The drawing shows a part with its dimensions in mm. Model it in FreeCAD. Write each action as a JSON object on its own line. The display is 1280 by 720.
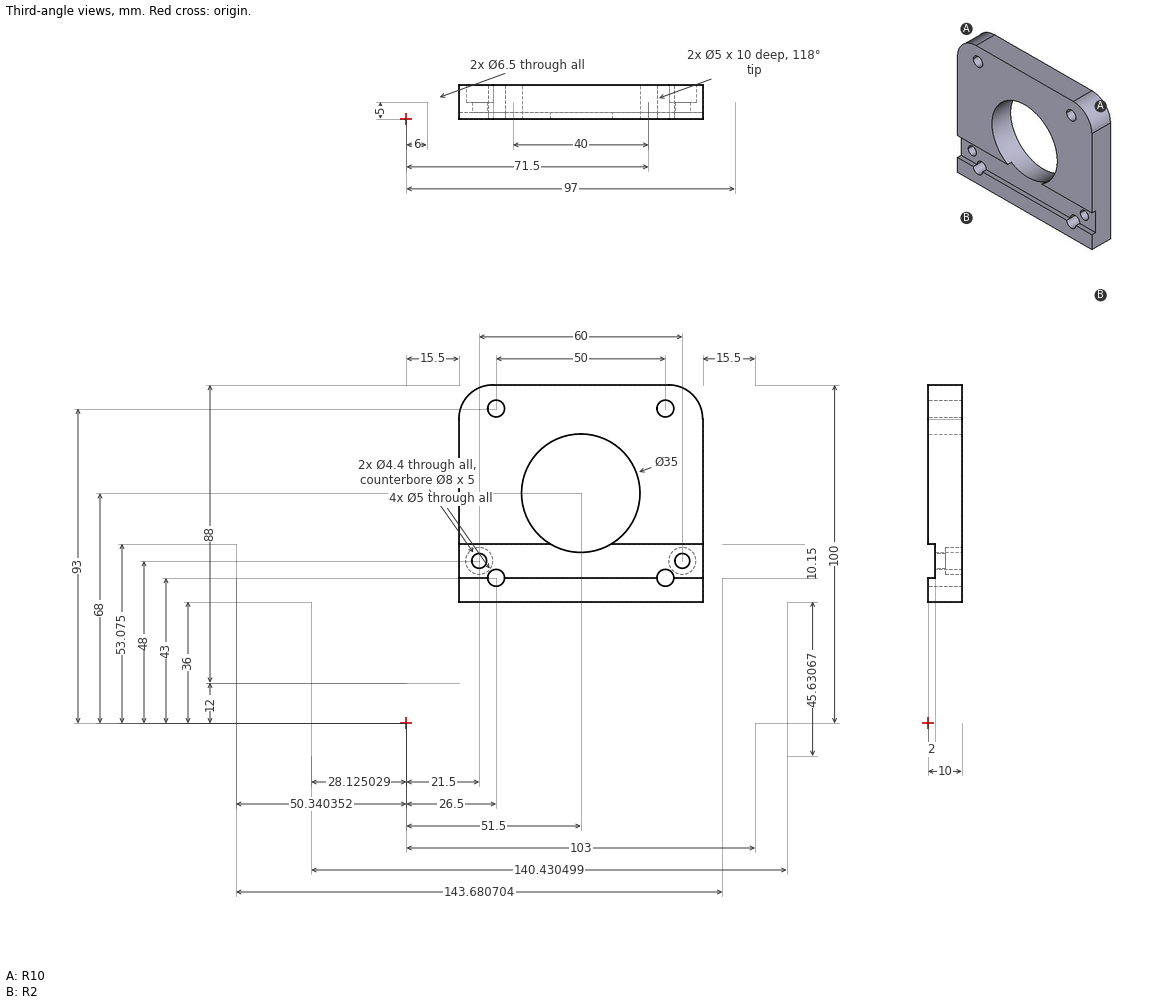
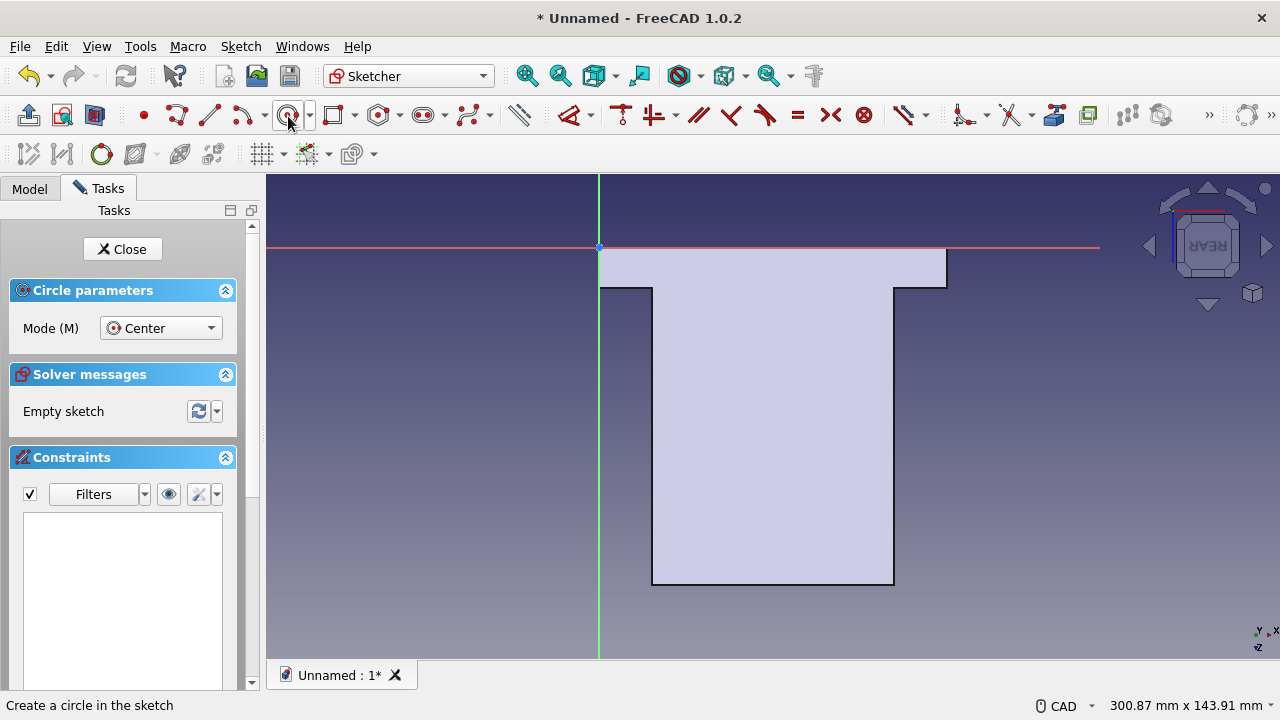
{"action": "left_click", "coordinate": [773, 477]}
{"action": "mouse_move", "coordinate": [815, 435]}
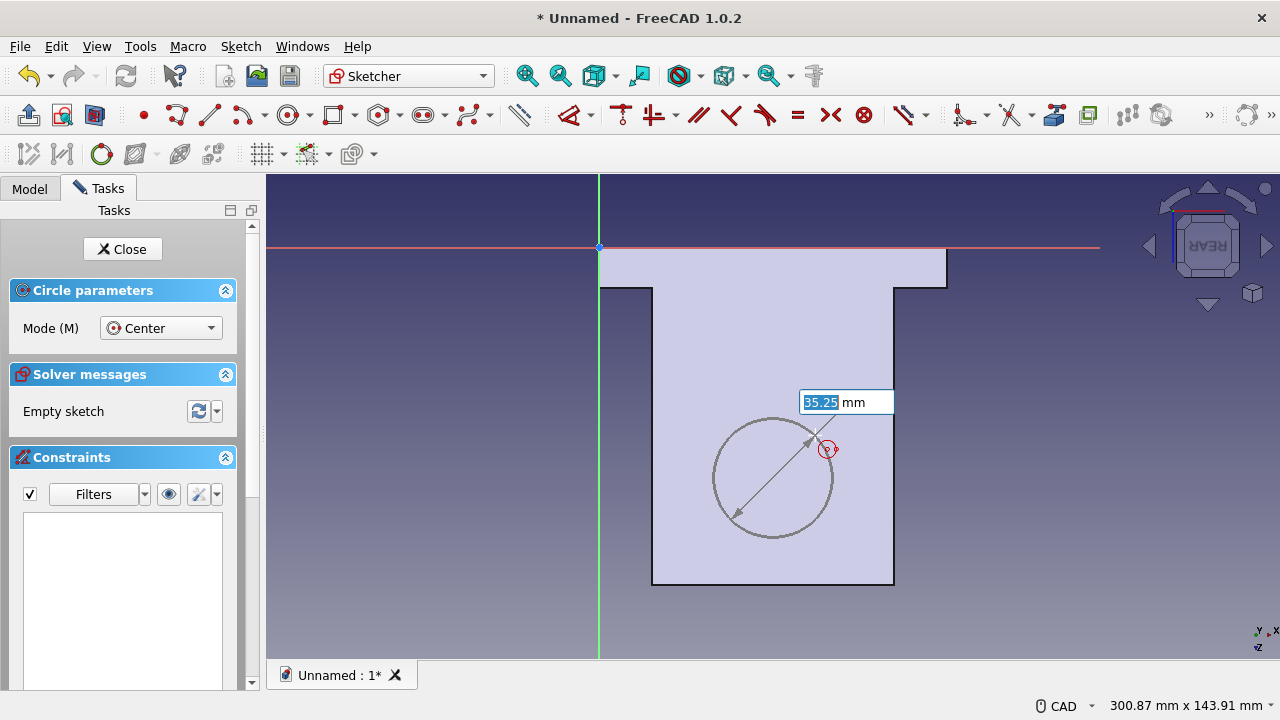
{"action": "type", "text": "35"}
{"action": "key", "text": "Return"}
{"action": "key", "text": "Escape"}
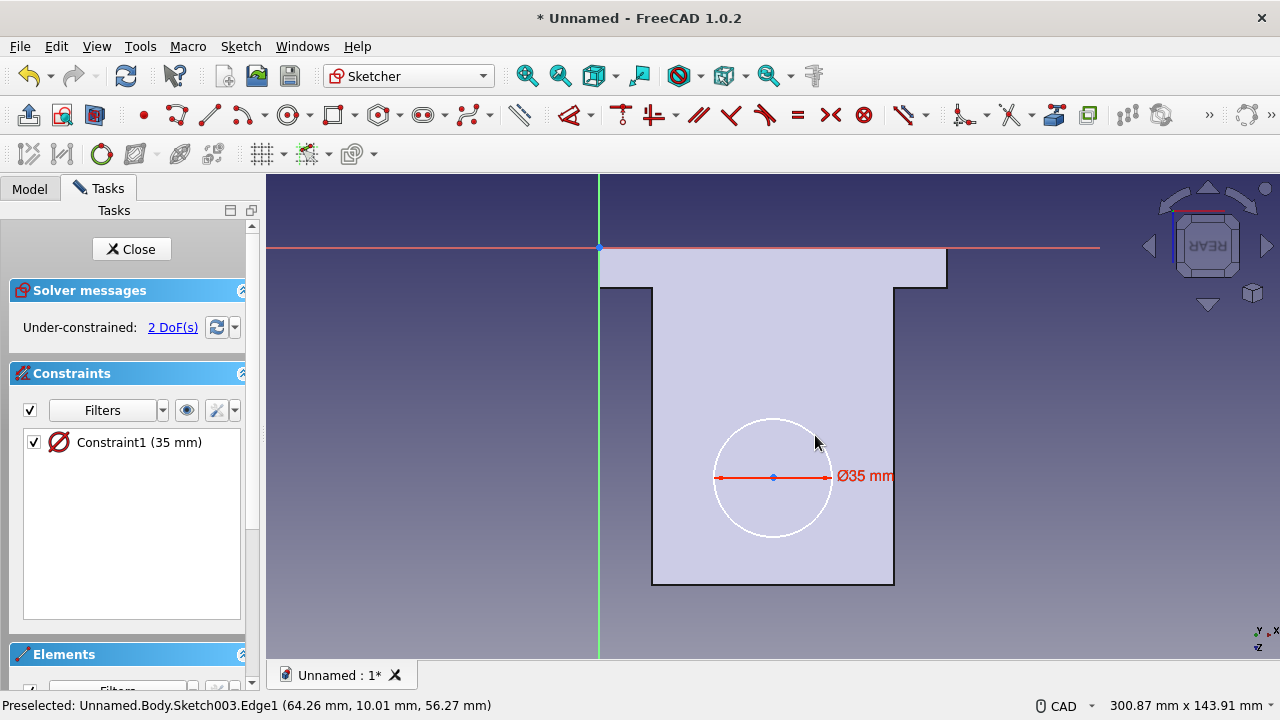
{"action": "left_click", "coordinate": [568, 116]}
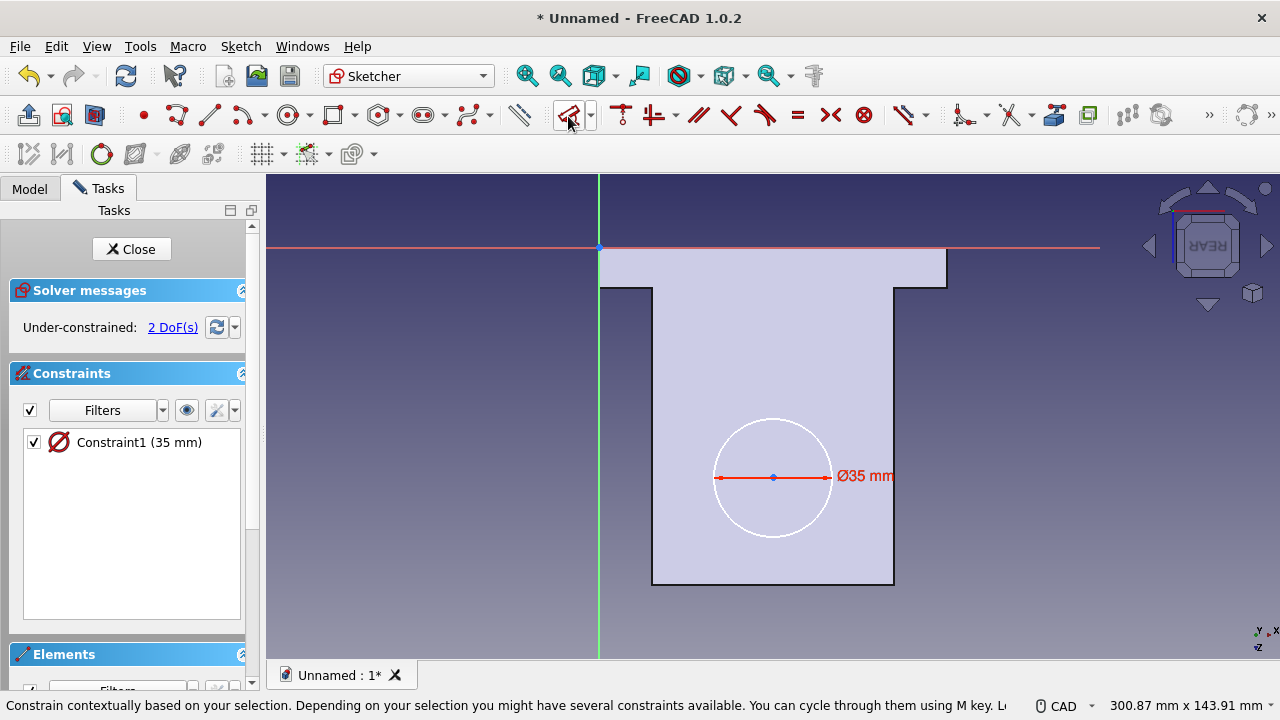
{"action": "left_click", "coordinate": [773, 478]}
{"action": "left_click", "coordinate": [565, 363]}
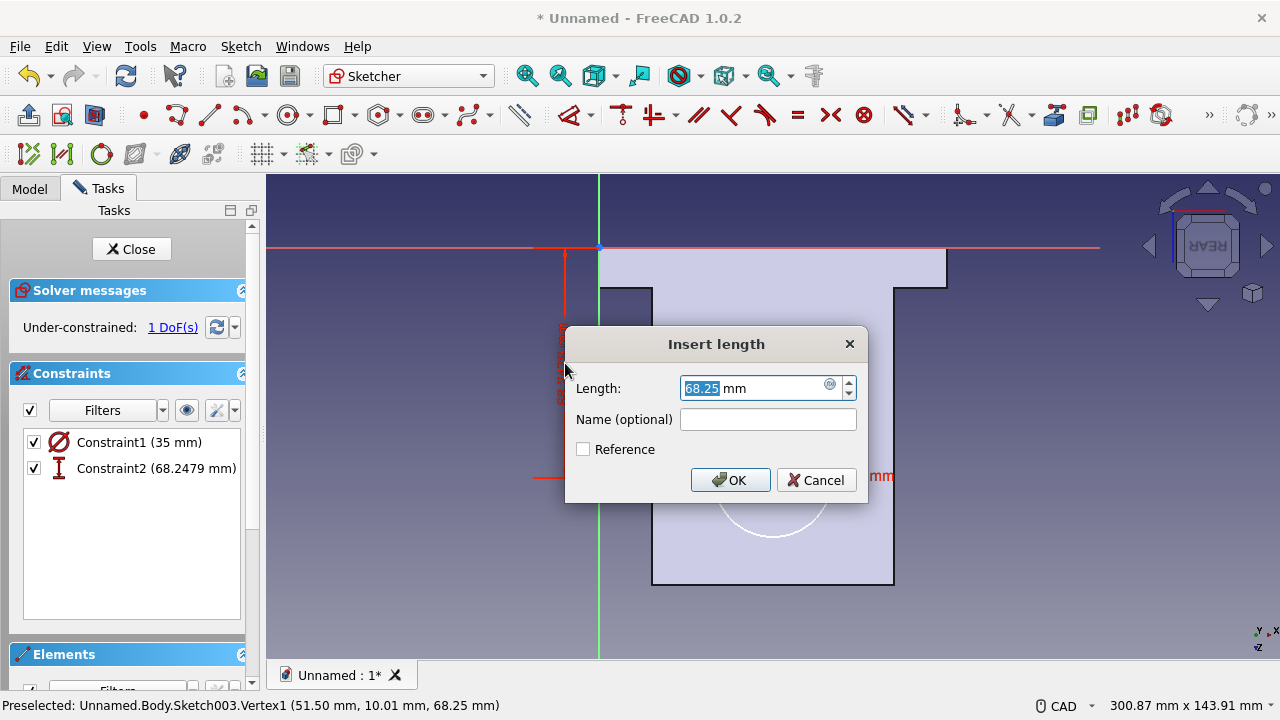
{"action": "type", "text": "68"}
{"action": "key", "text": "Return"}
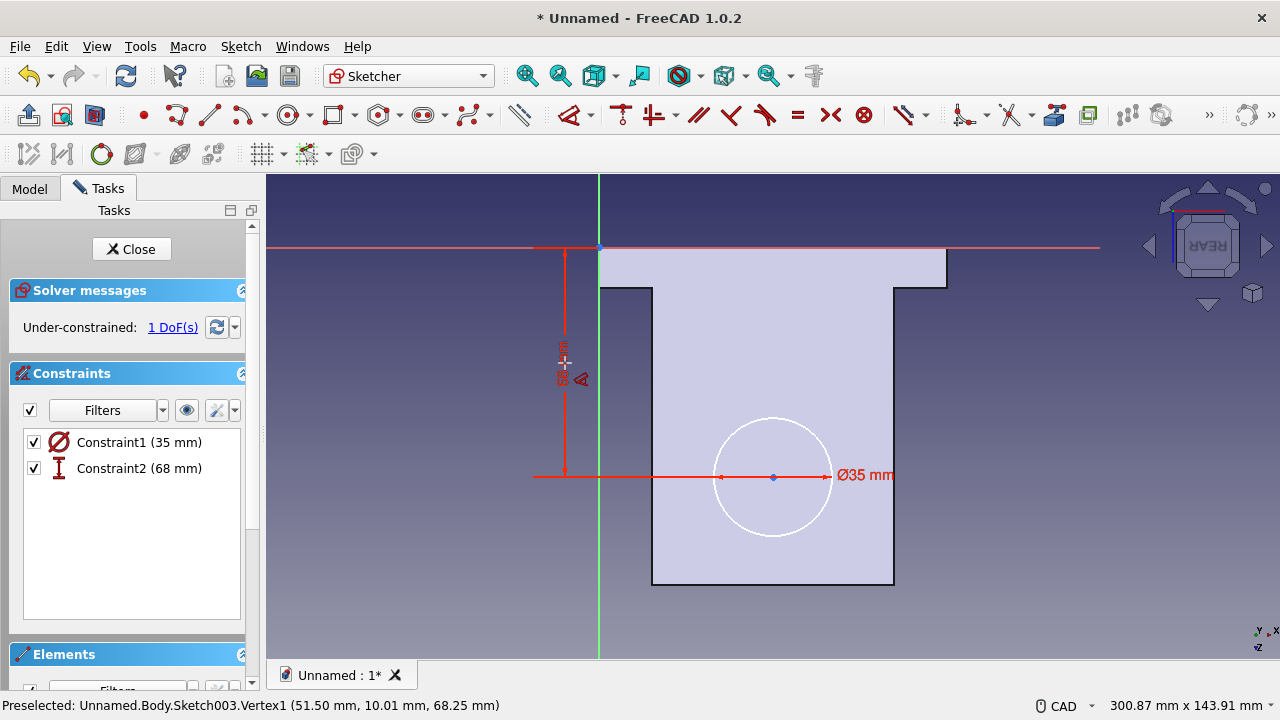
{"action": "left_click", "coordinate": [773, 477]}
{"action": "left_click", "coordinate": [686, 214]}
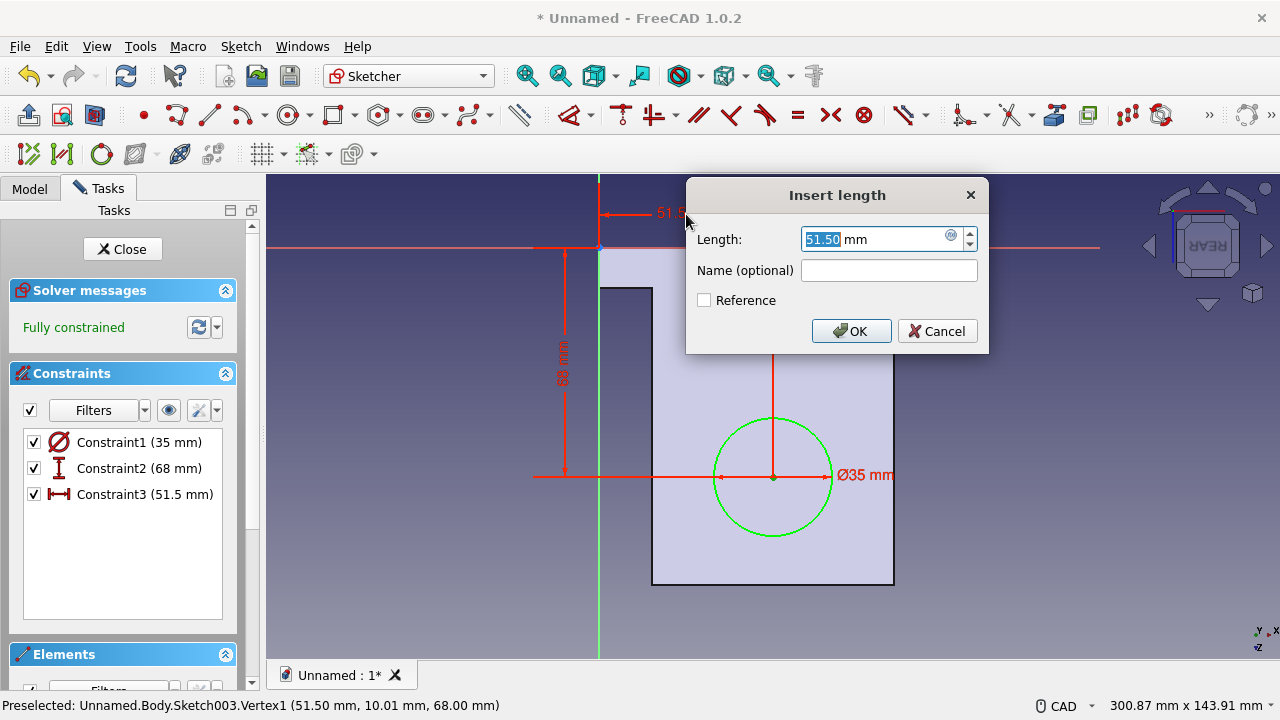
{"action": "type", "text": "51.5"}
{"action": "key", "text": "Return"}
{"action": "key", "text": "Escape"}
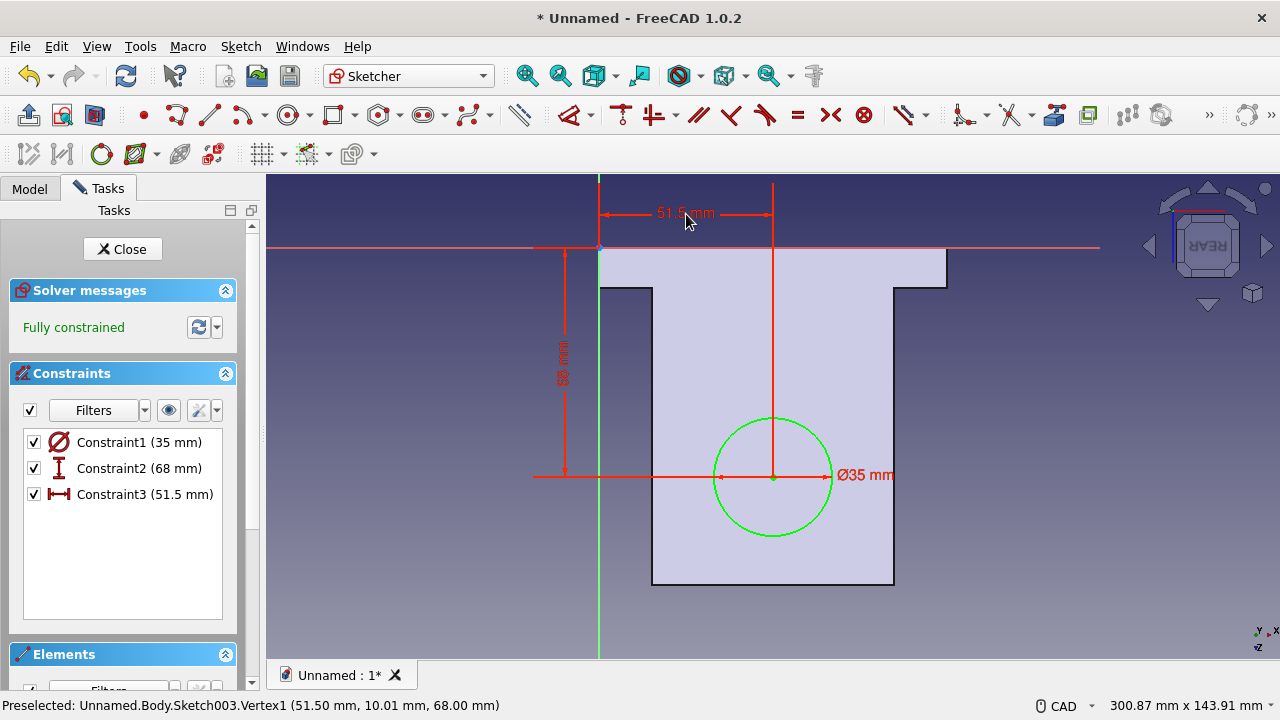
{"action": "left_click", "coordinate": [123, 249]}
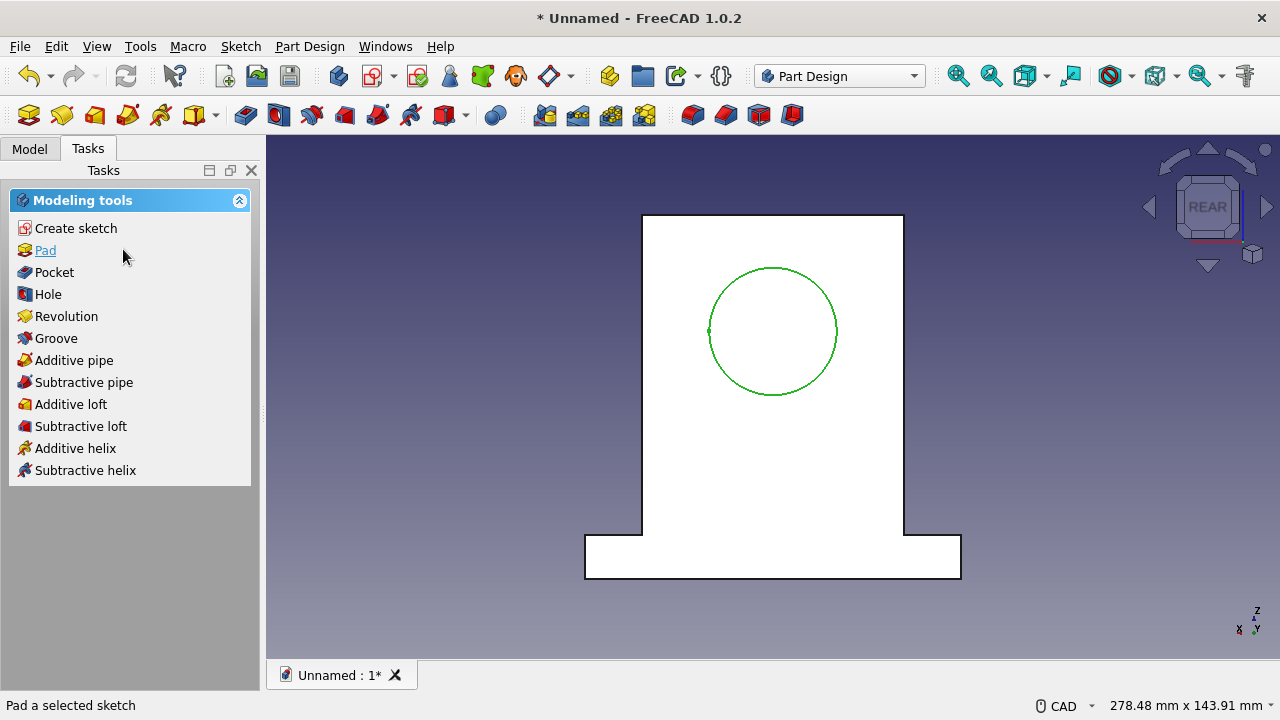
{"action": "left_click", "coordinate": [246, 116]}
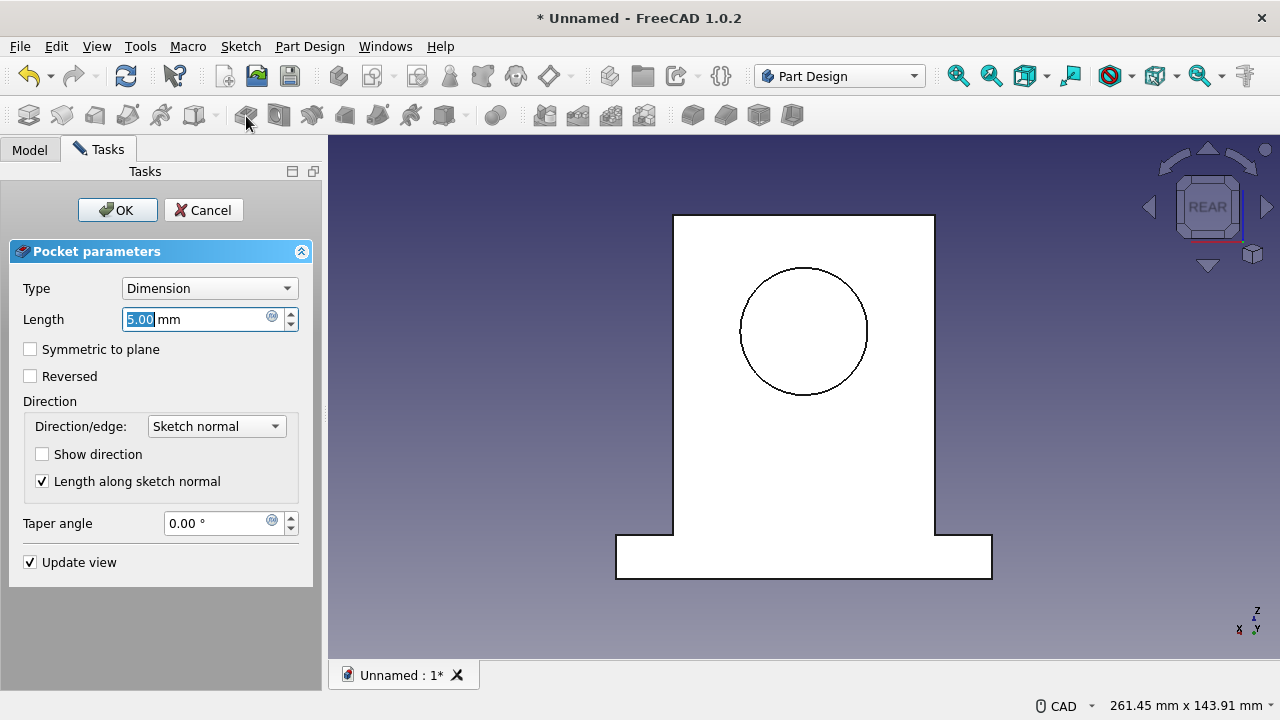
{"action": "left_click", "coordinate": [210, 288]}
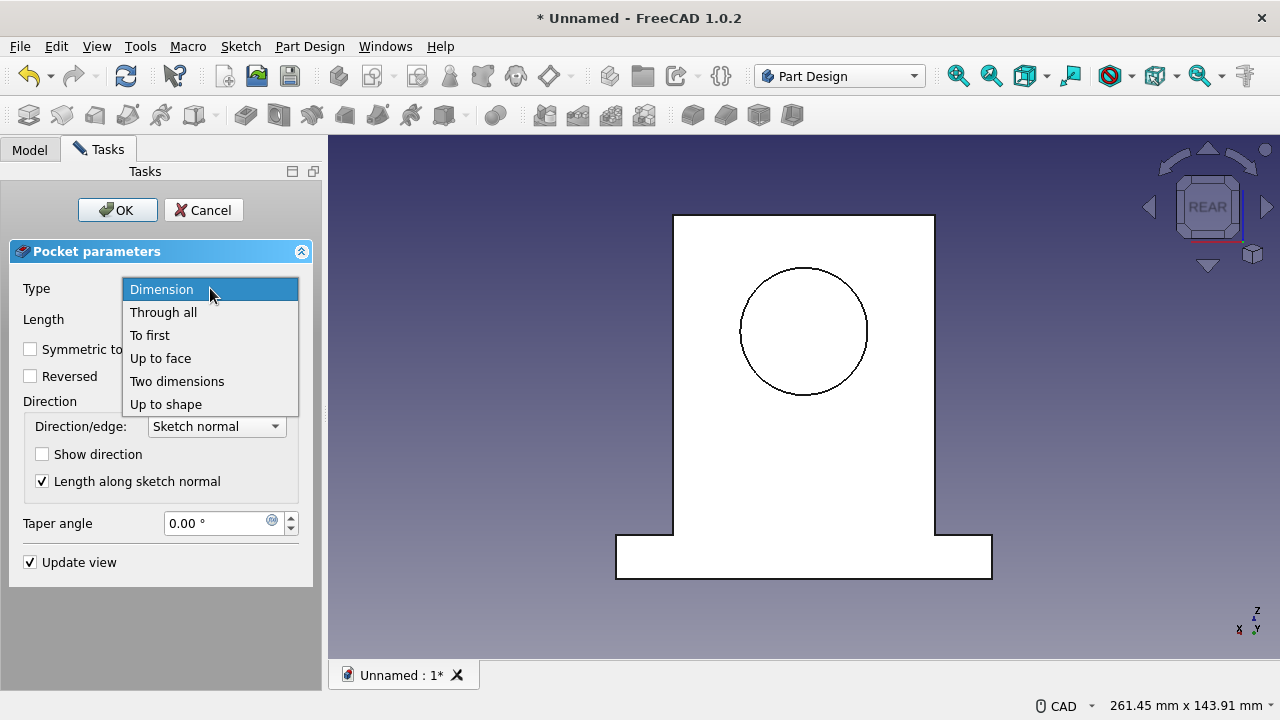
{"action": "left_click", "coordinate": [208, 312]}